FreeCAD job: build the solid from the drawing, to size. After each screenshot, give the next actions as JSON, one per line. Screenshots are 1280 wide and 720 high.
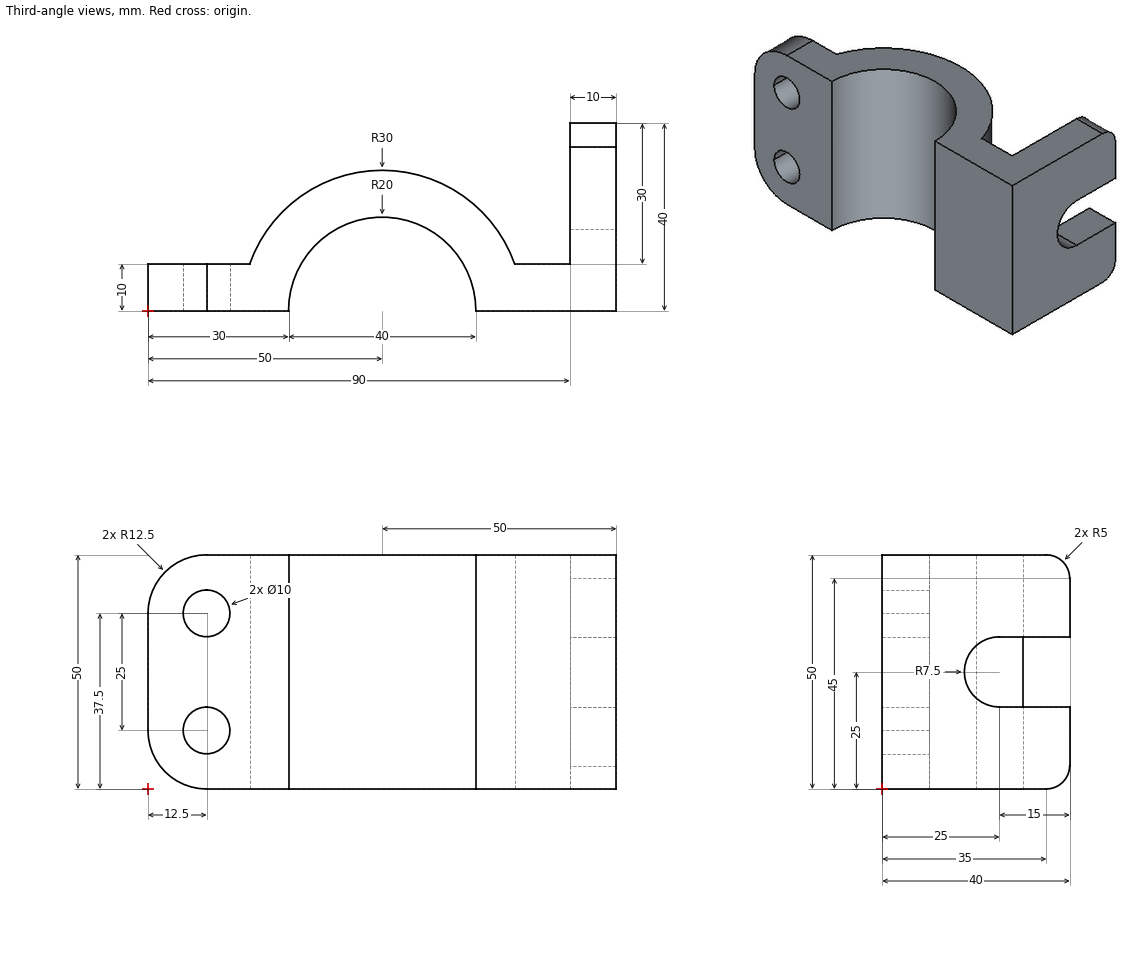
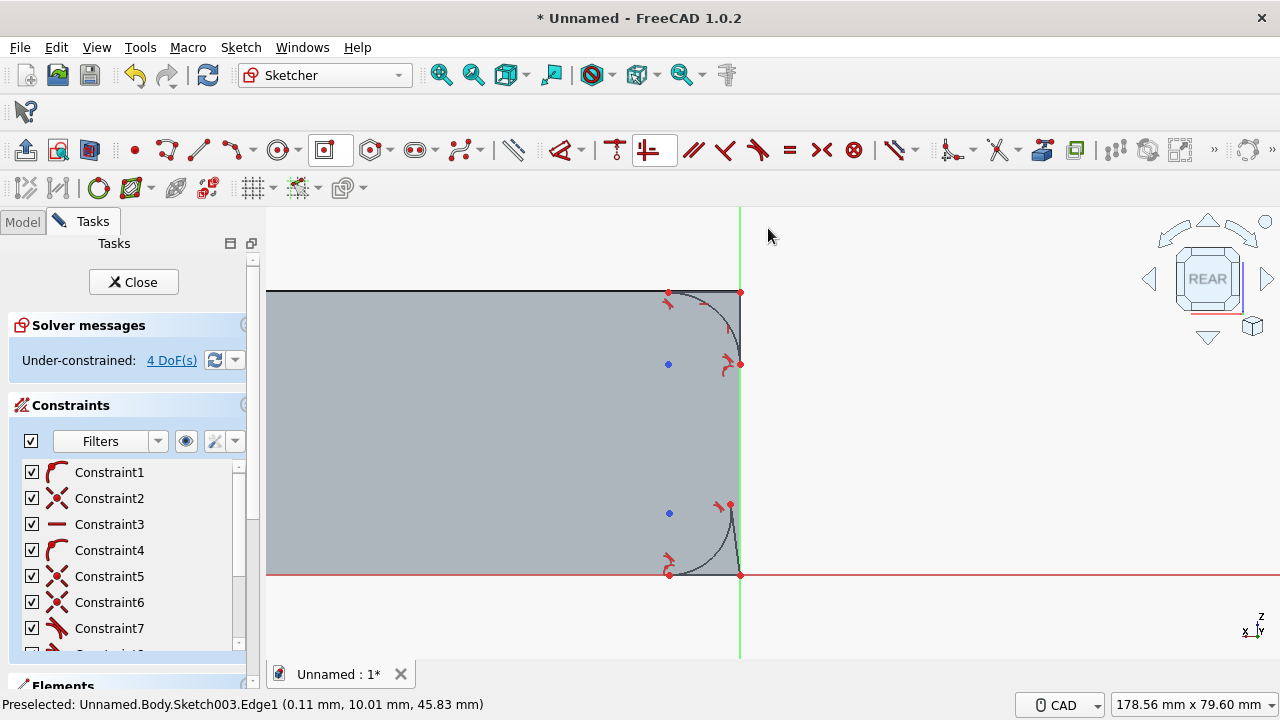
{"action": "left_click", "coordinate": [737, 554]}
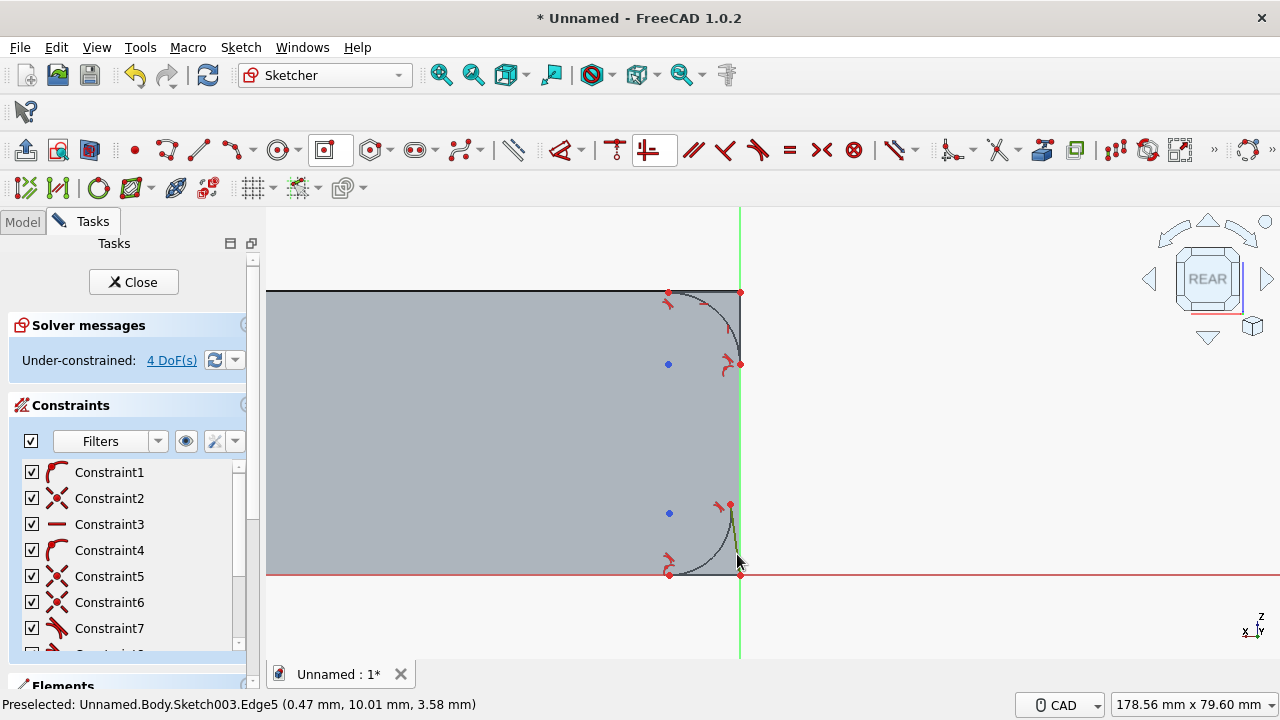
{"action": "left_click", "coordinate": [672, 150]}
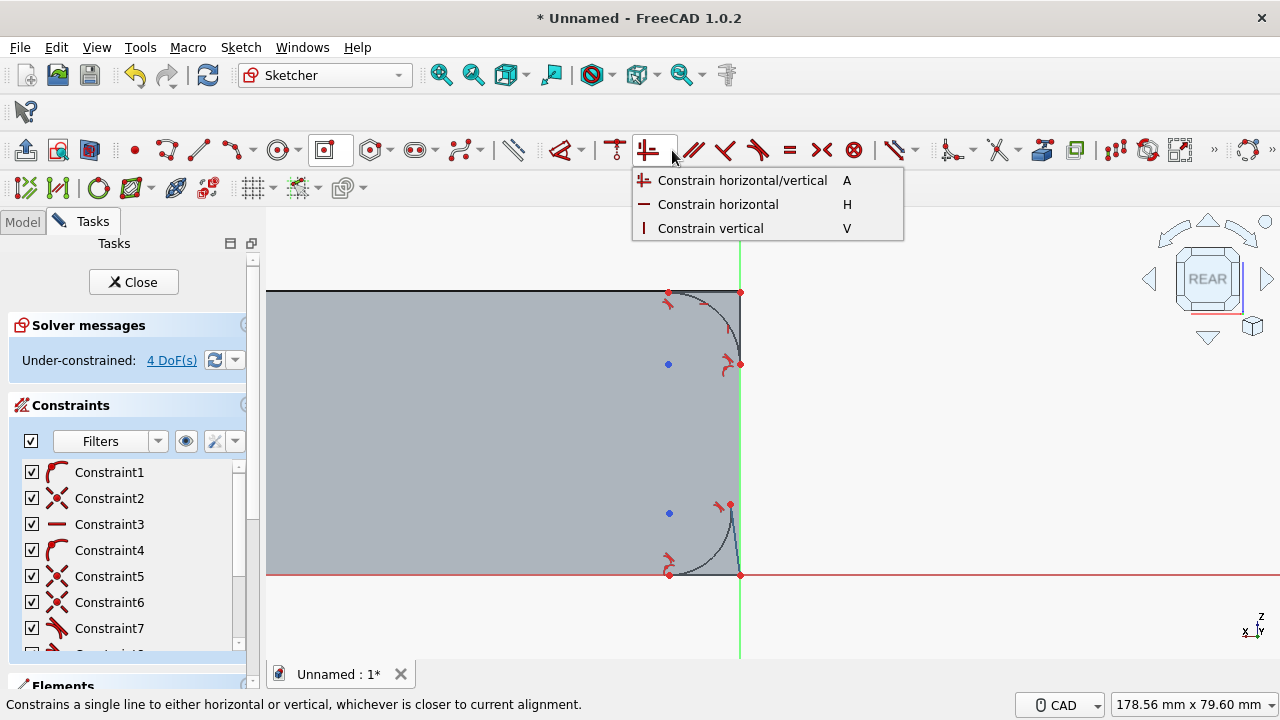
{"action": "left_click", "coordinate": [768, 228]}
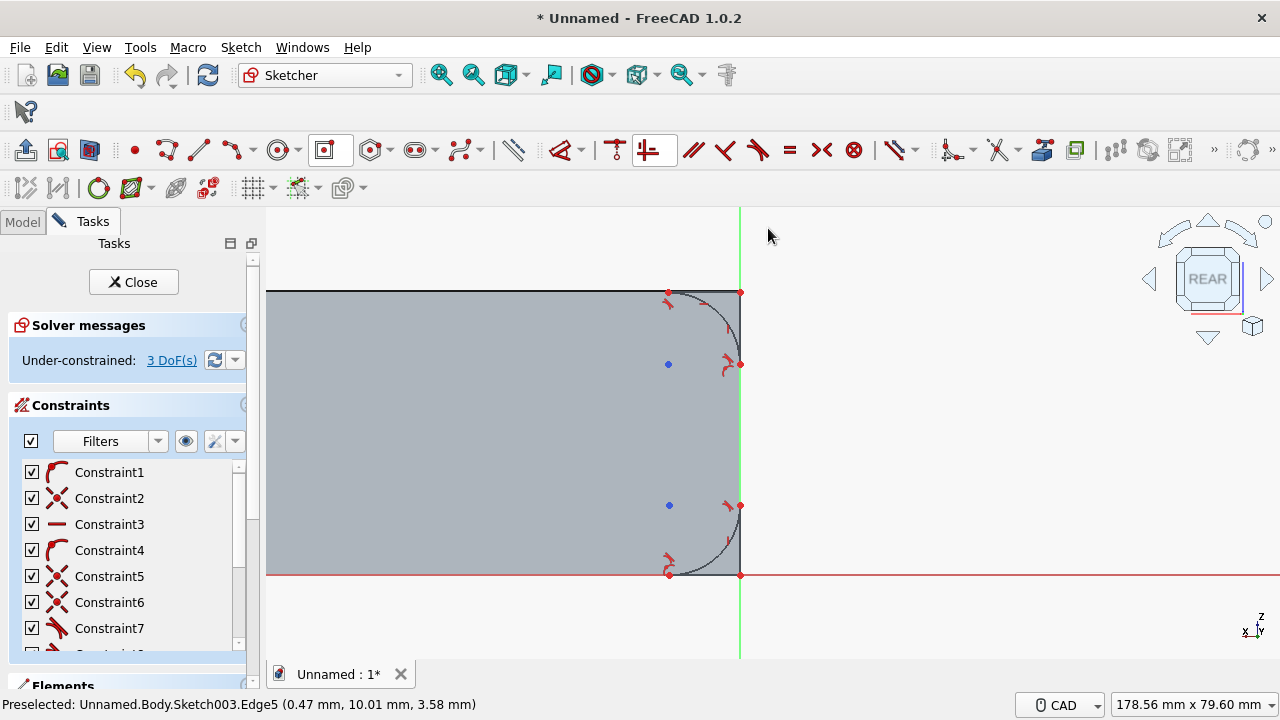
{"action": "left_click", "coordinate": [719, 313]}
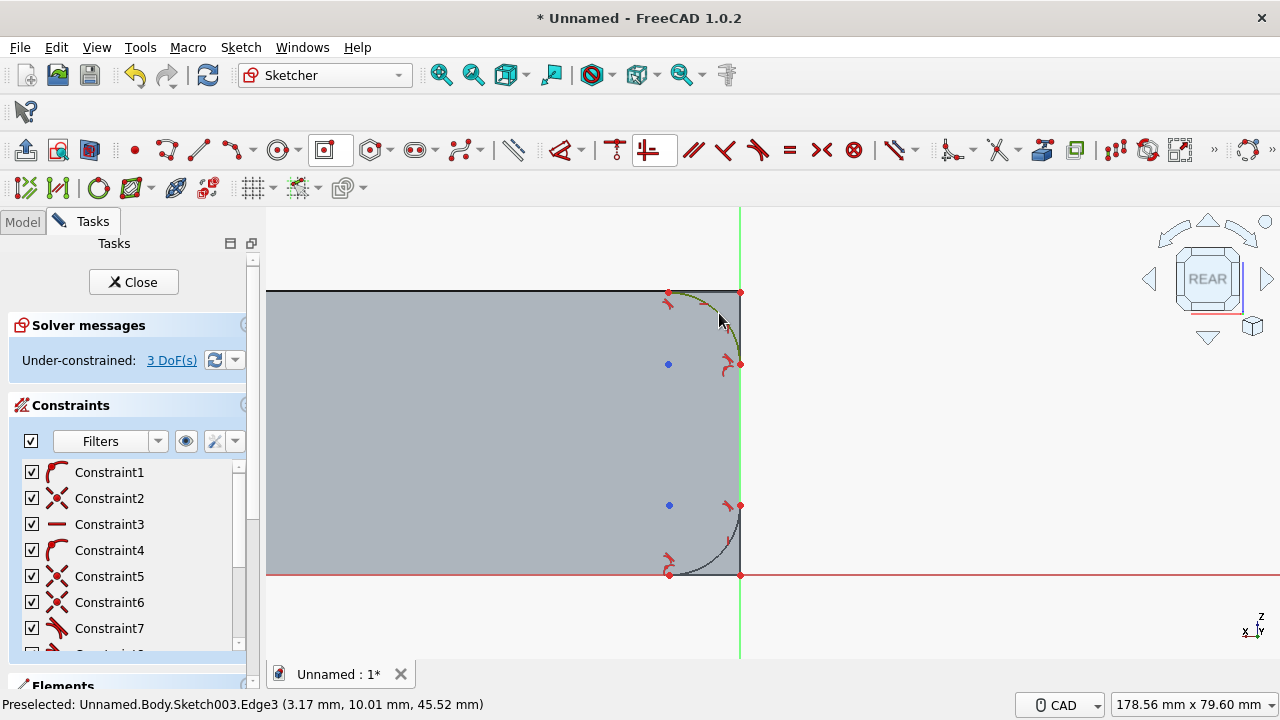
{"action": "left_click", "coordinate": [719, 555]}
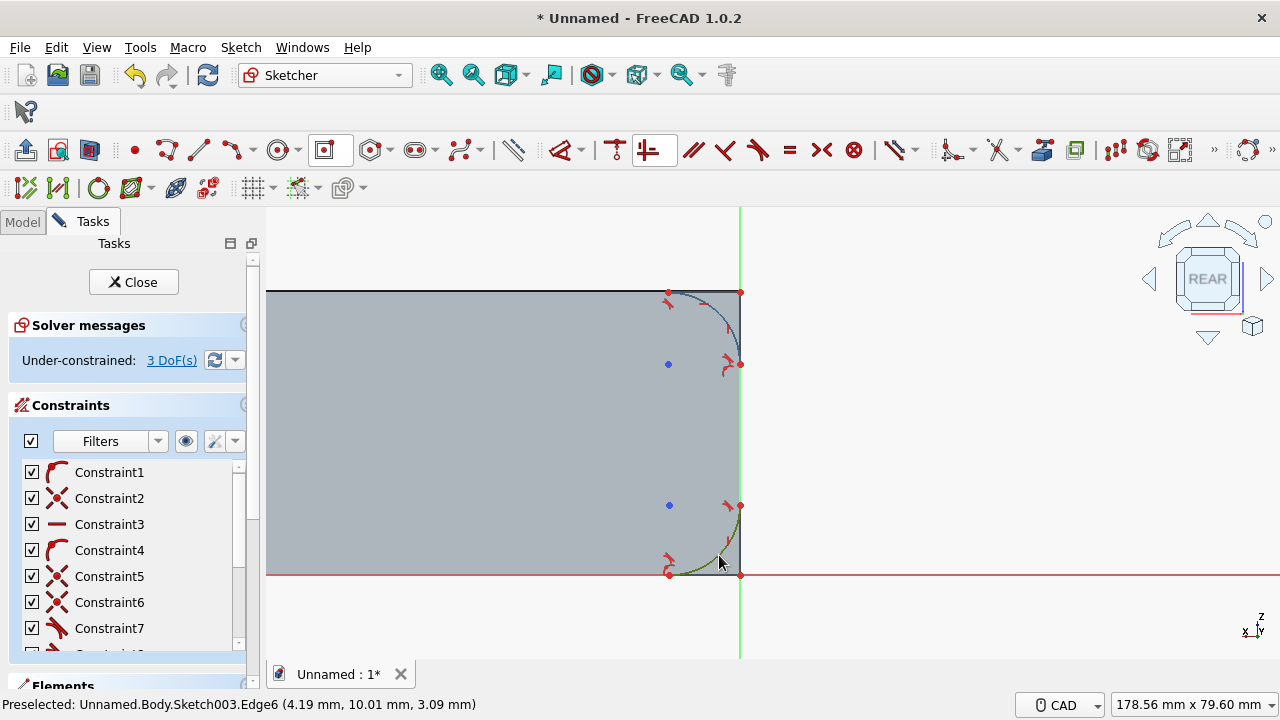
{"action": "left_click", "coordinate": [790, 150]}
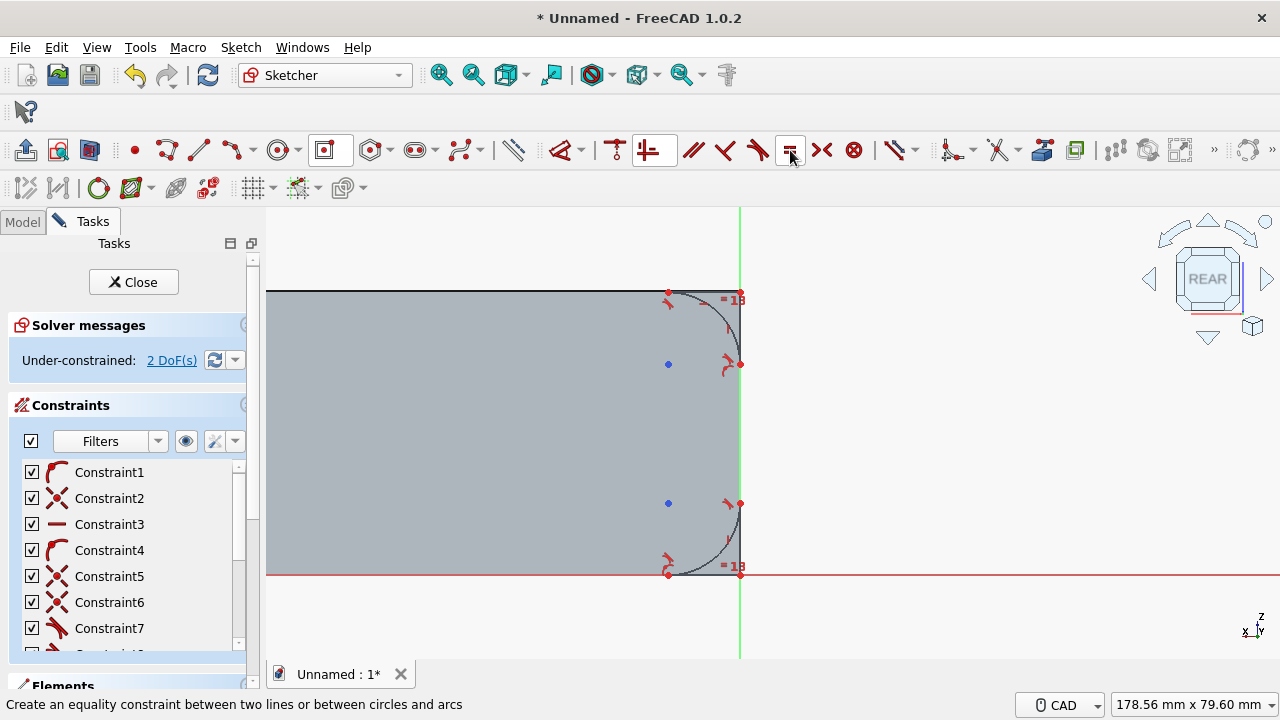
{"action": "left_click", "coordinate": [560, 150]}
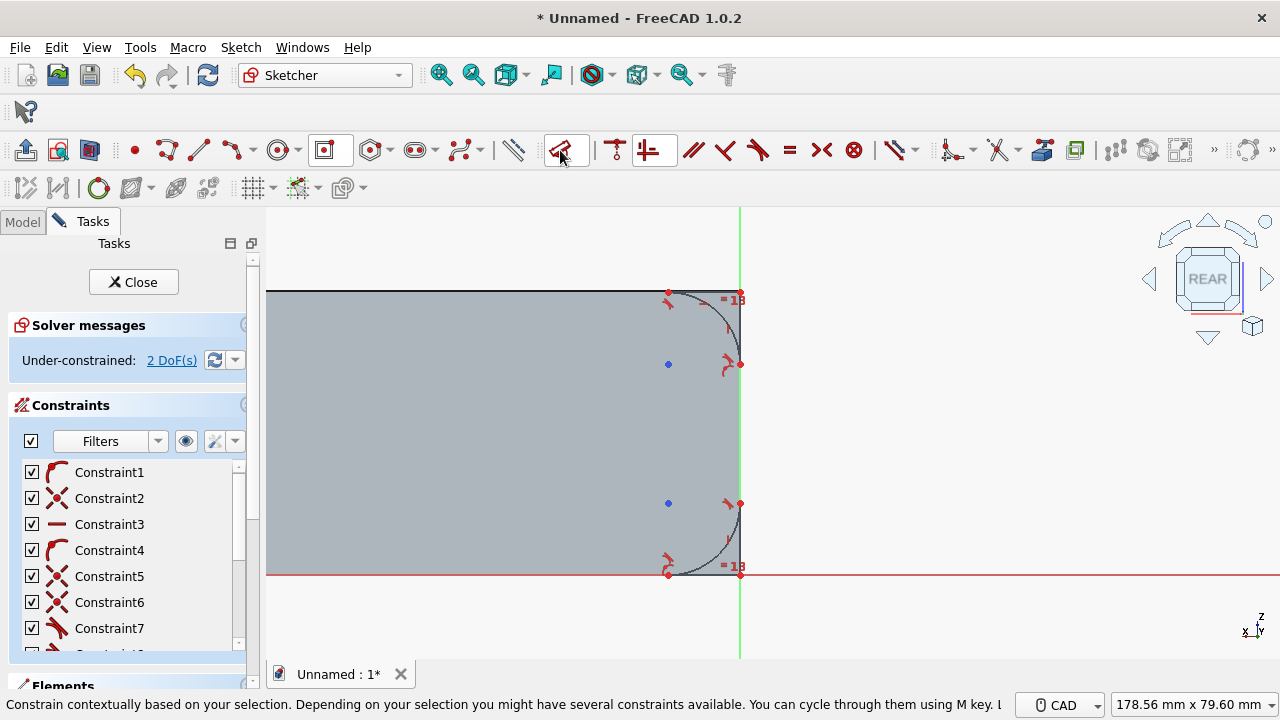
{"action": "left_click", "coordinate": [719, 313]}
{"action": "left_click", "coordinate": [768, 335]}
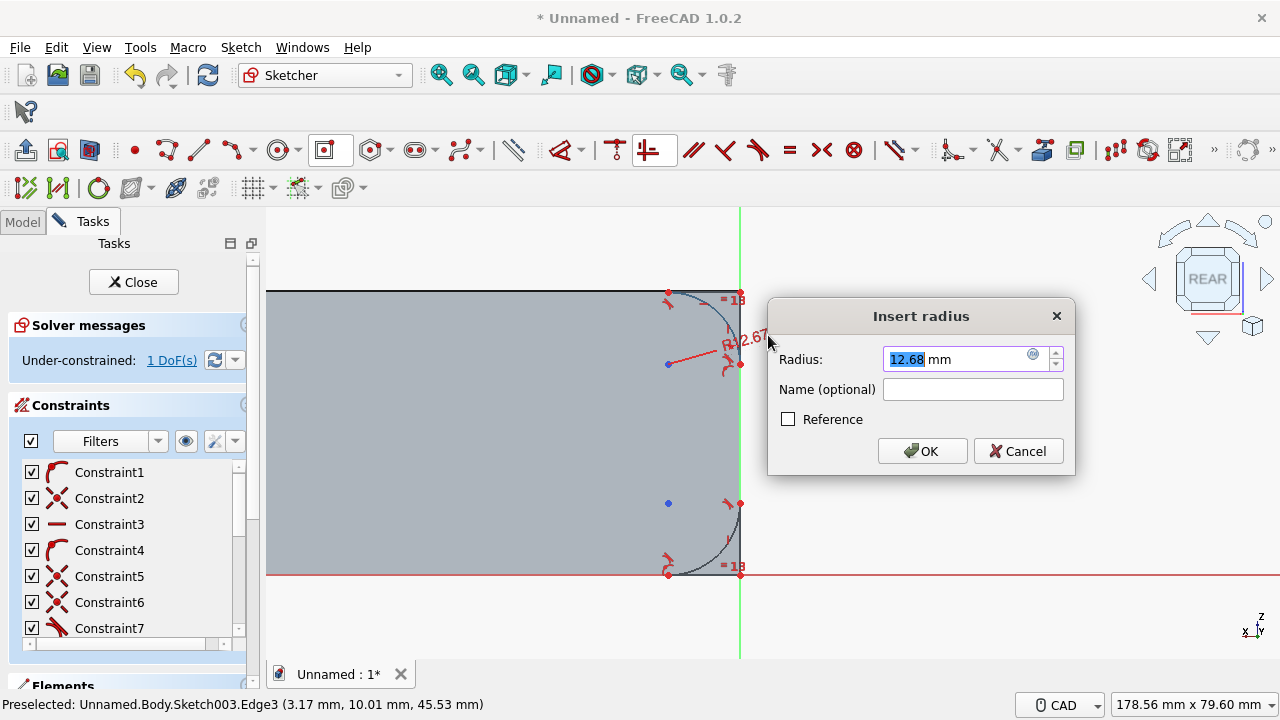
{"action": "type", "text": "12.5"}
{"action": "key", "text": "Return"}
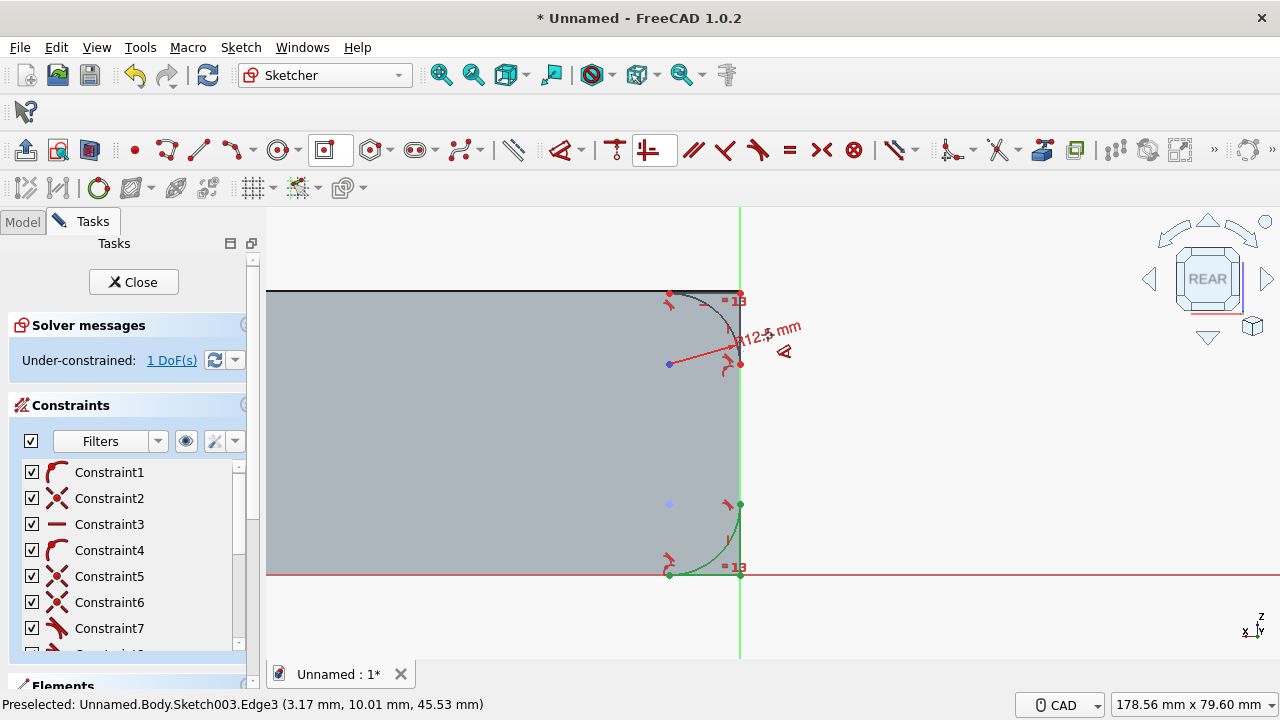
{"action": "left_click", "coordinate": [740, 293]}
{"action": "left_click", "coordinate": [774, 434]}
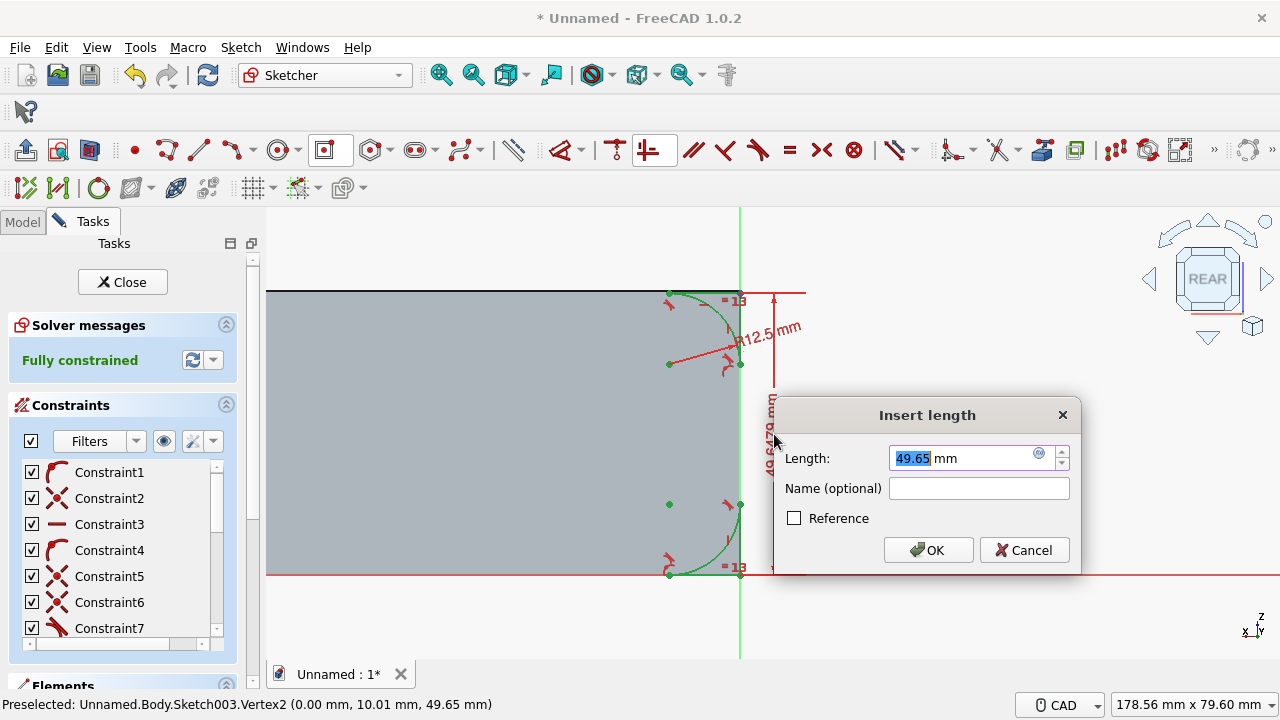
{"action": "type", "text": "50"}
{"action": "key", "text": "Return"}
{"action": "key", "text": "Escape"}